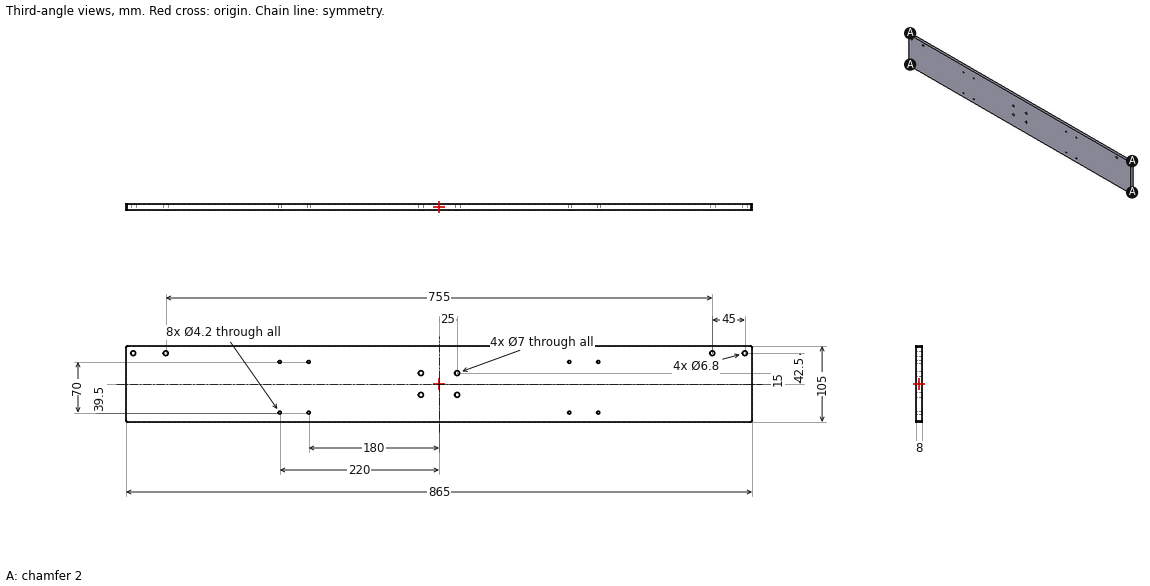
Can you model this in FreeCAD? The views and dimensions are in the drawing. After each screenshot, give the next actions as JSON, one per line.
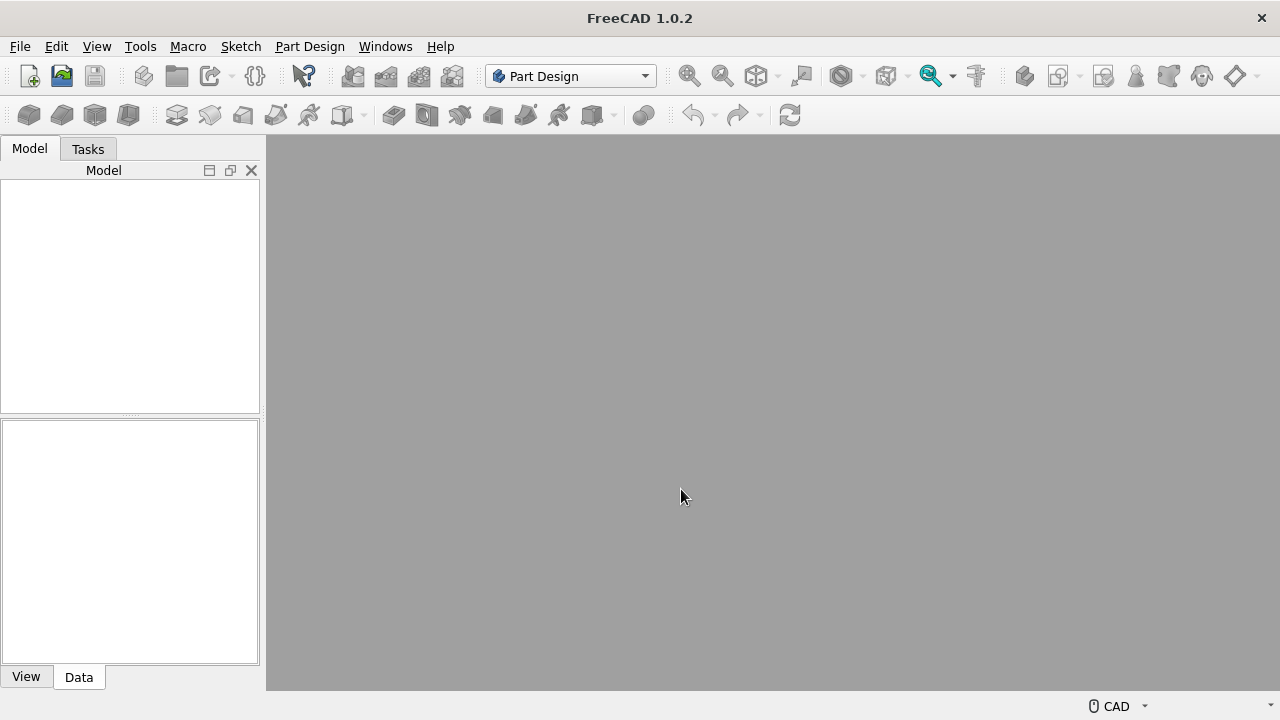
{"action": "key", "text": "ctrl+n"}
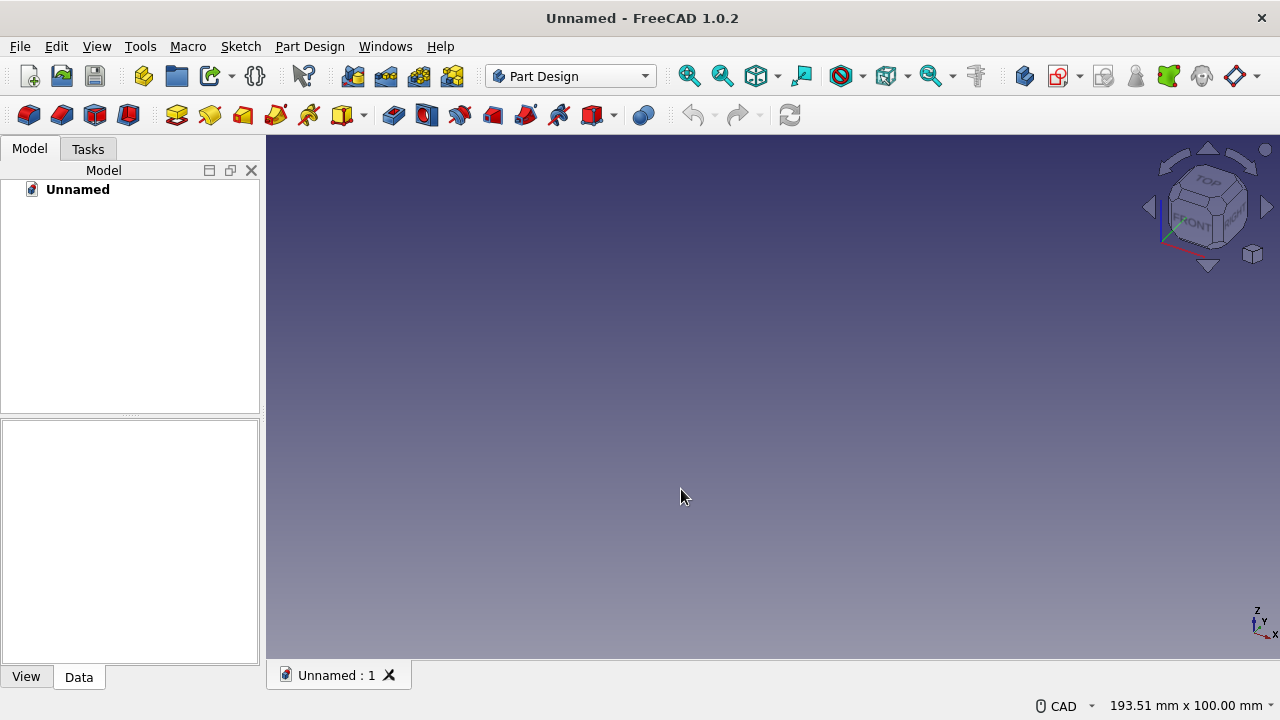
{"action": "left_click", "coordinate": [1058, 76]}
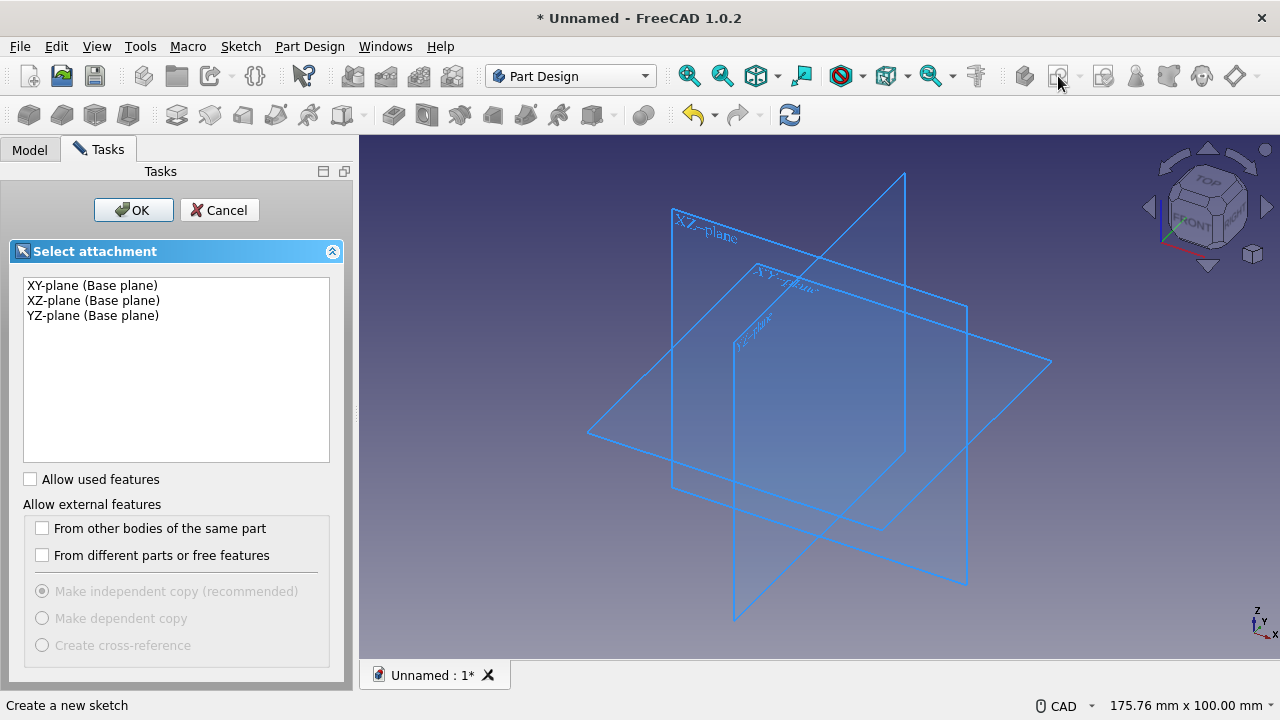
{"action": "left_click", "coordinate": [84, 300]}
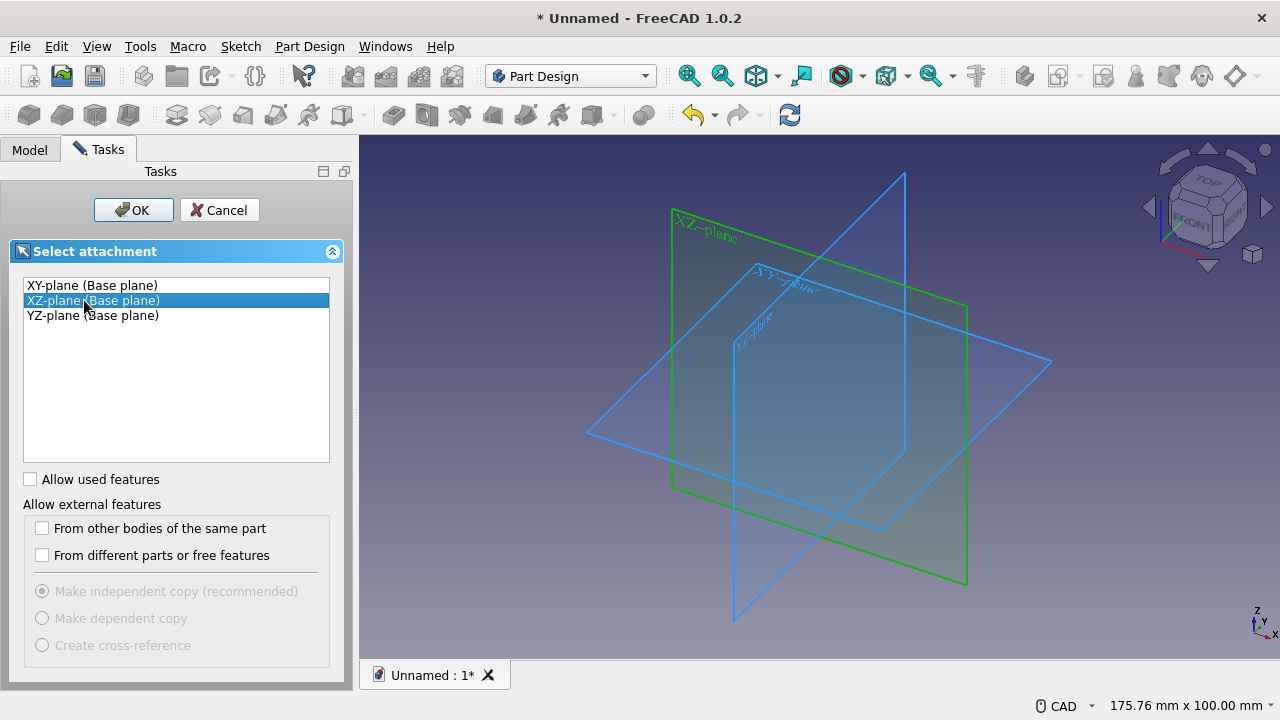
{"action": "left_click", "coordinate": [134, 210]}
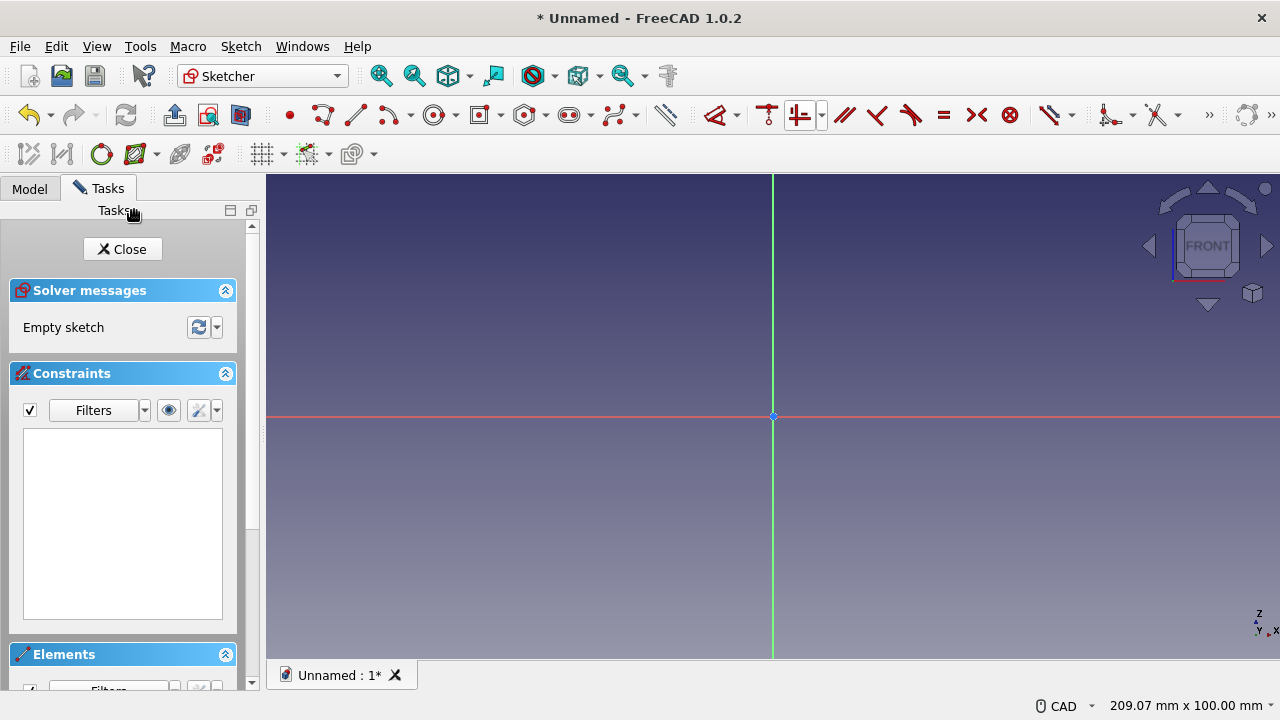
{"action": "scroll", "coordinate": [694, 416], "scroll_direction": "down", "scroll_amount": 10}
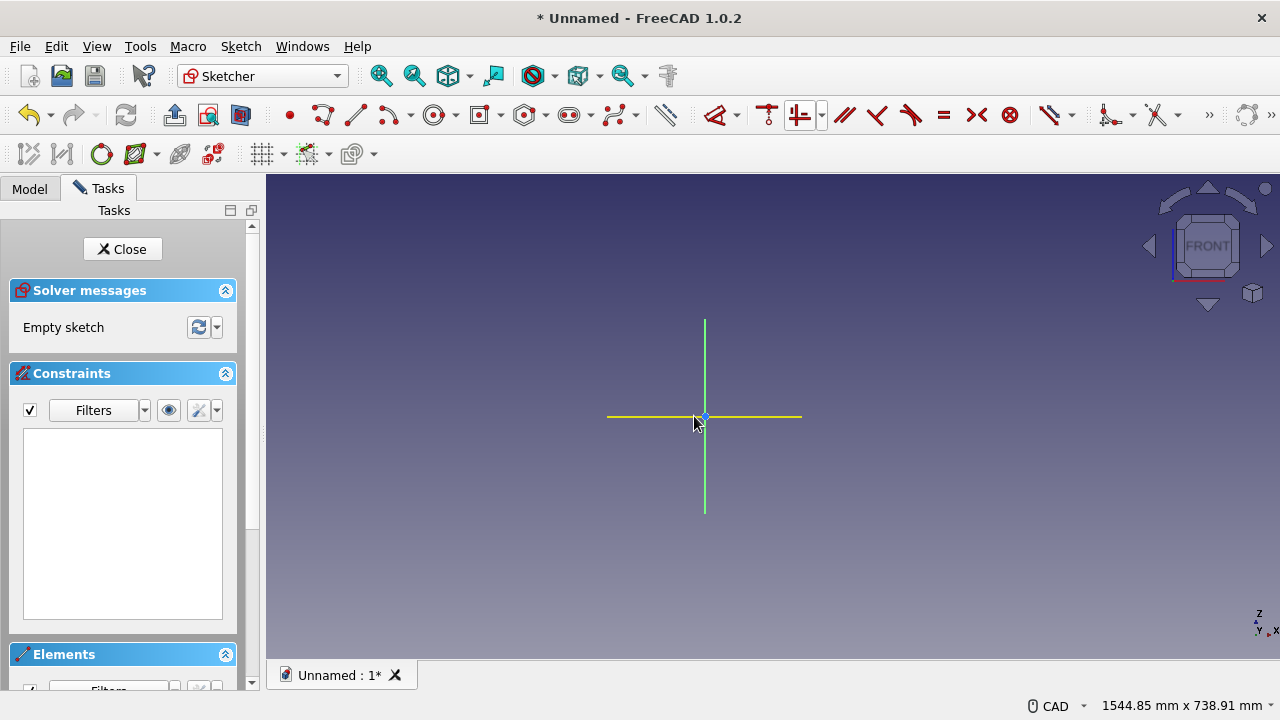
{"action": "left_click", "coordinate": [478, 116]}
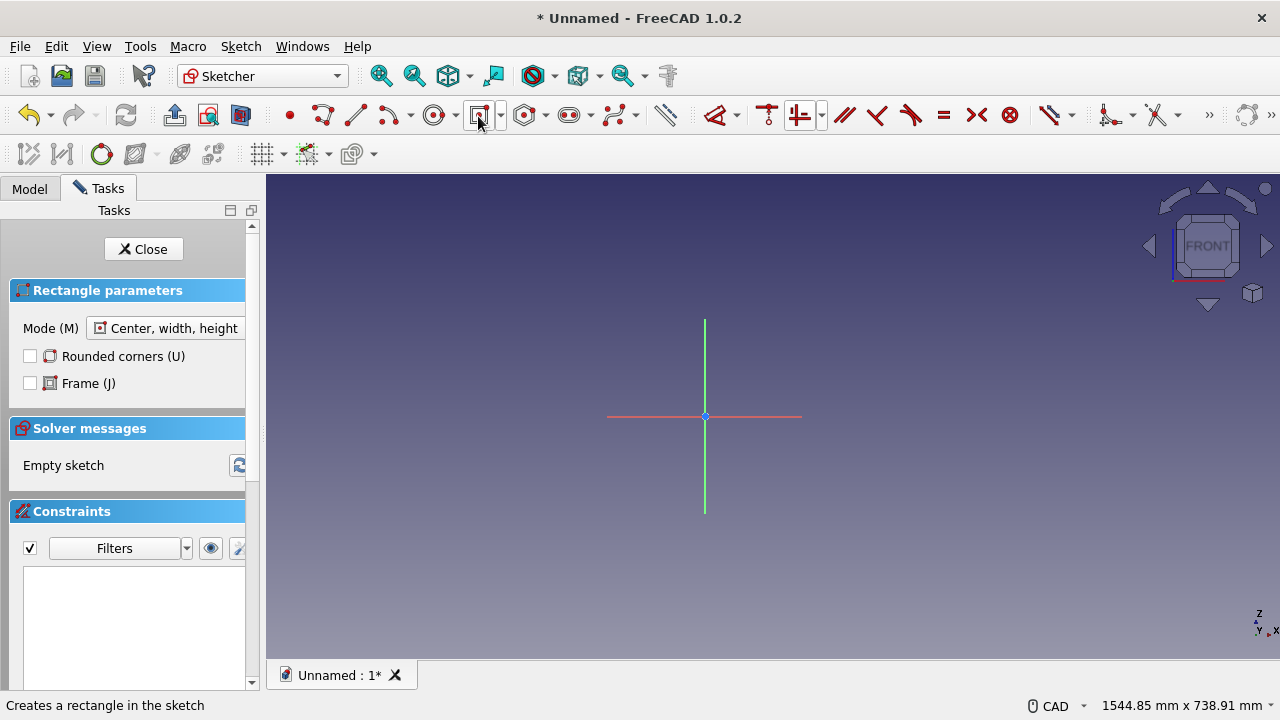
{"action": "left_click", "coordinate": [705, 416]}
{"action": "left_click", "coordinate": [989, 382]}
{"action": "key", "text": "Escape"}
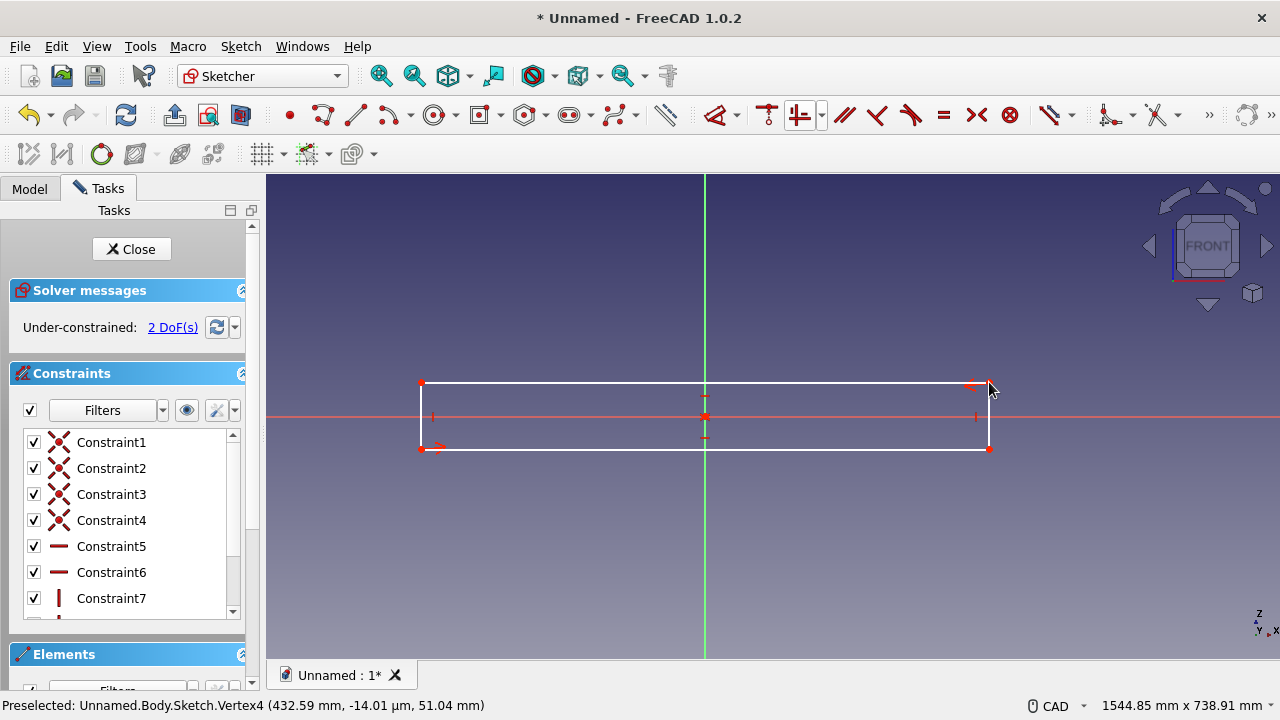
{"action": "key", "text": "d"}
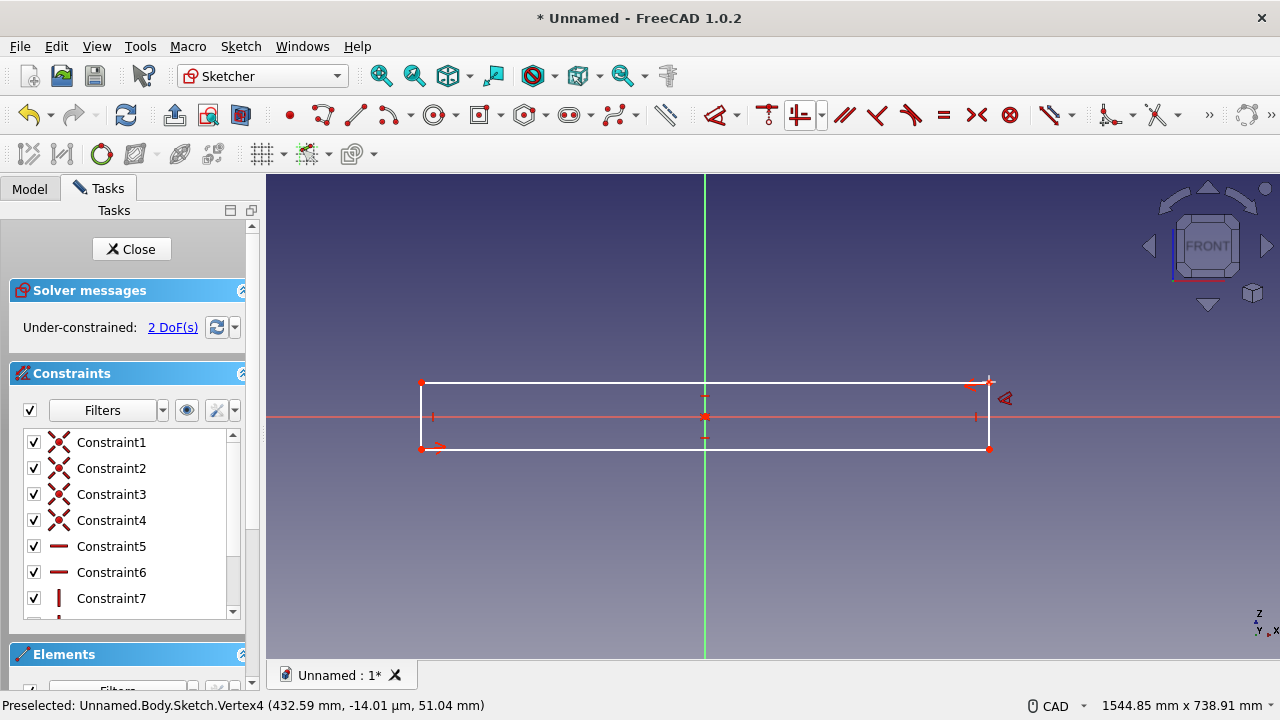
{"action": "left_click", "coordinate": [591, 450]}
{"action": "left_click", "coordinate": [574, 484]}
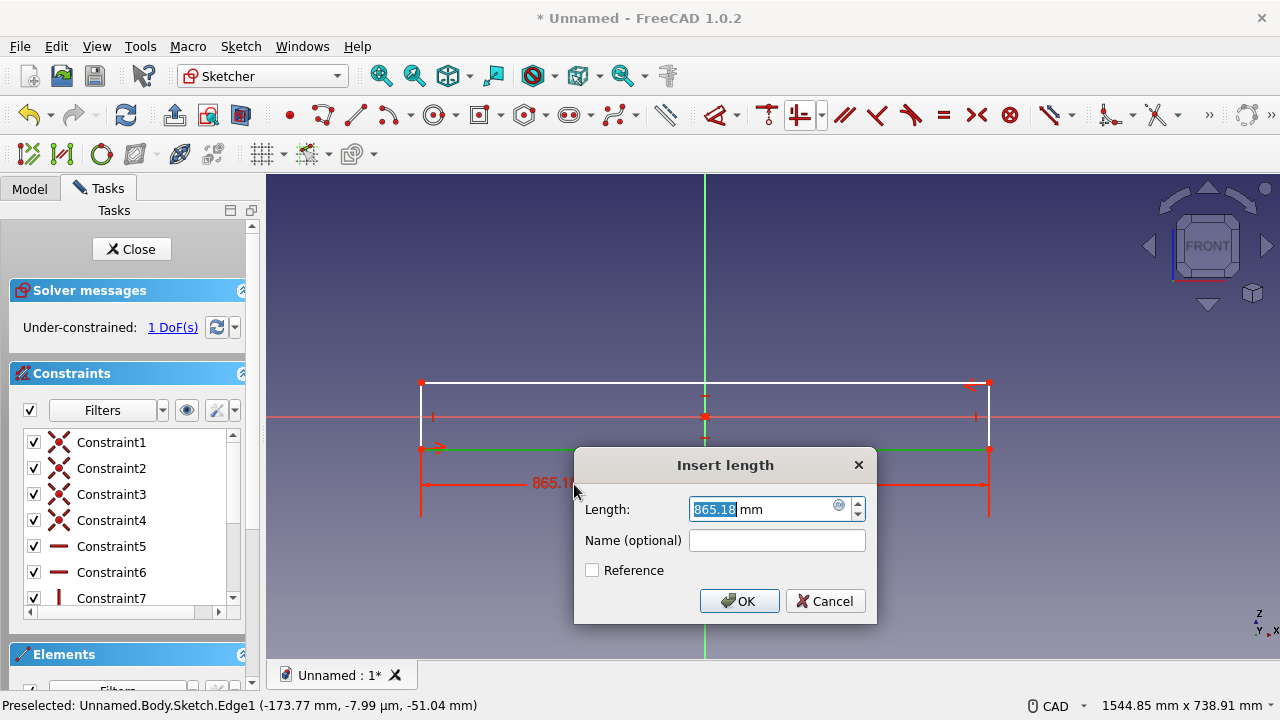
{"action": "type", "text": "865"}
{"action": "key", "text": "Return"}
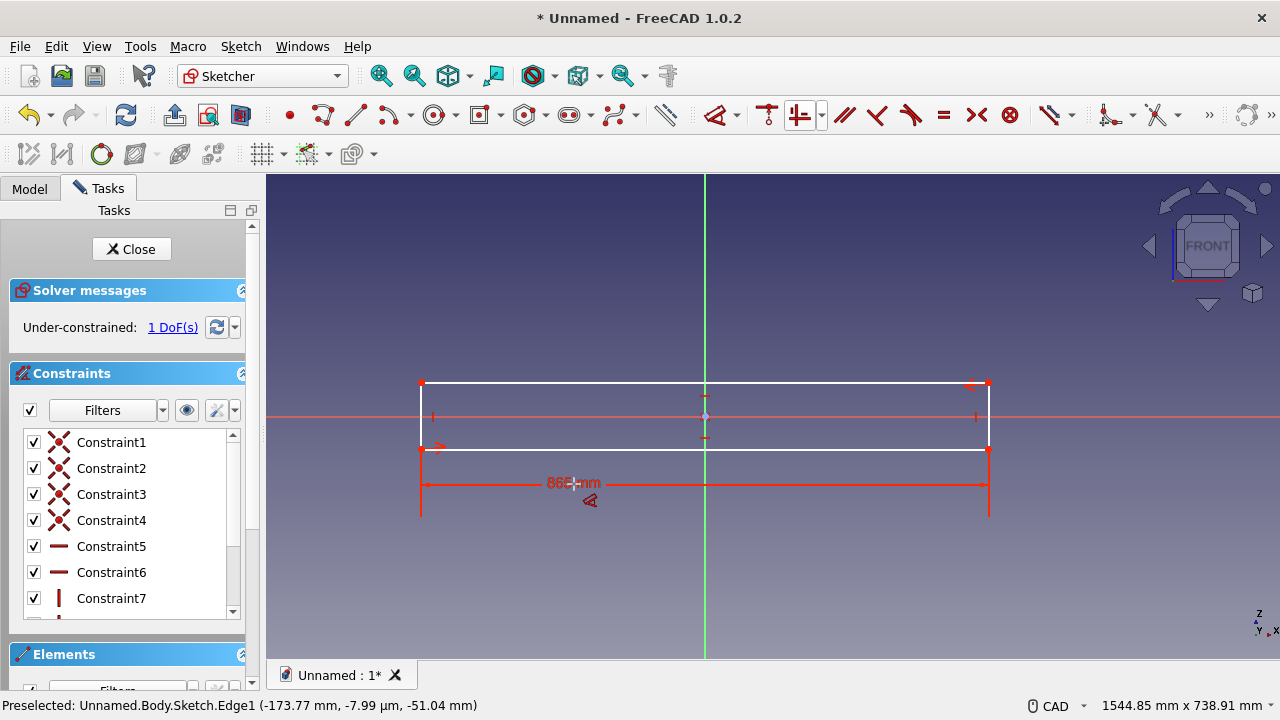
{"action": "left_click", "coordinate": [989, 430]}
{"action": "left_click", "coordinate": [1023, 401]}